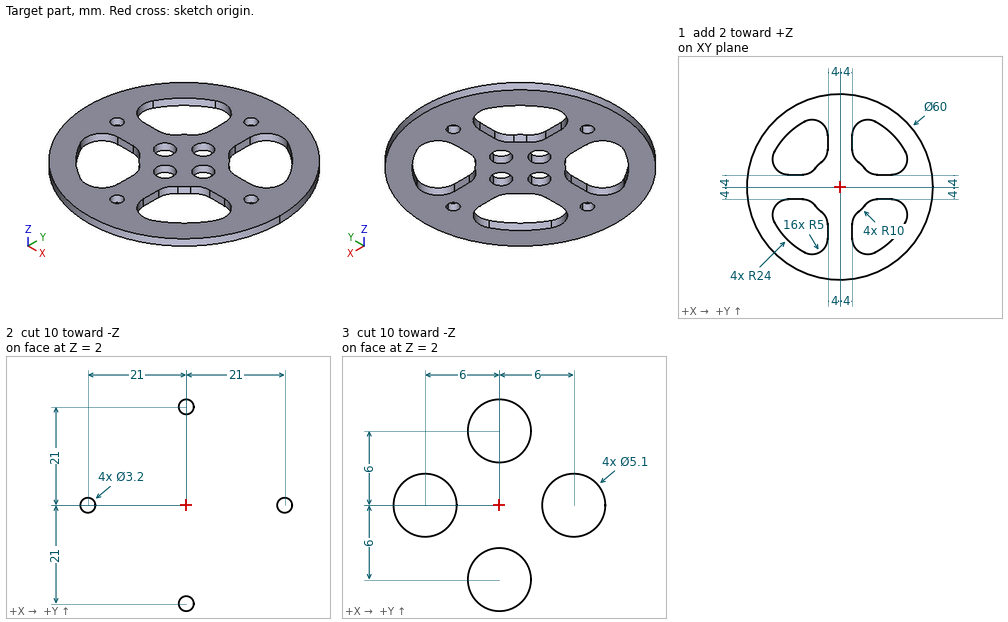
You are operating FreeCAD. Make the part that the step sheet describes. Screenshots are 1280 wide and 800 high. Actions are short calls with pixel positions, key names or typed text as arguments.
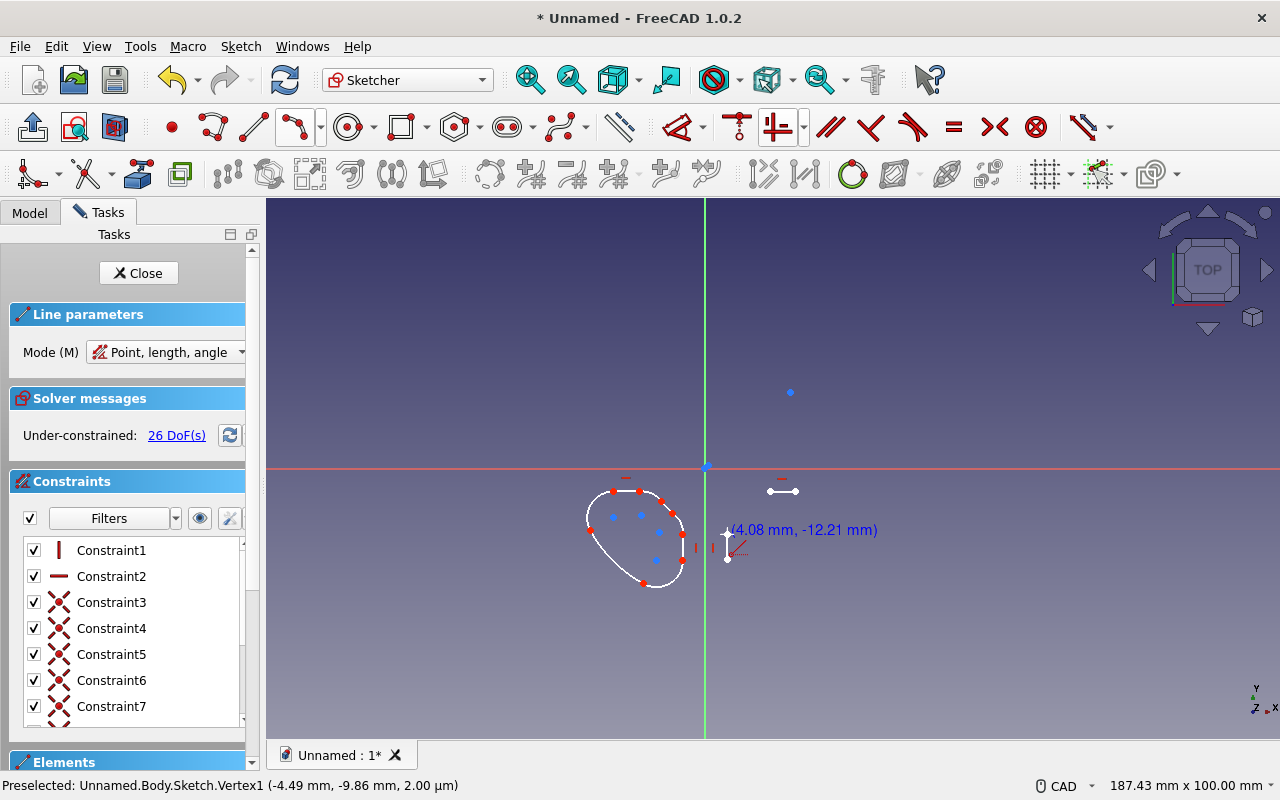
click(294, 128)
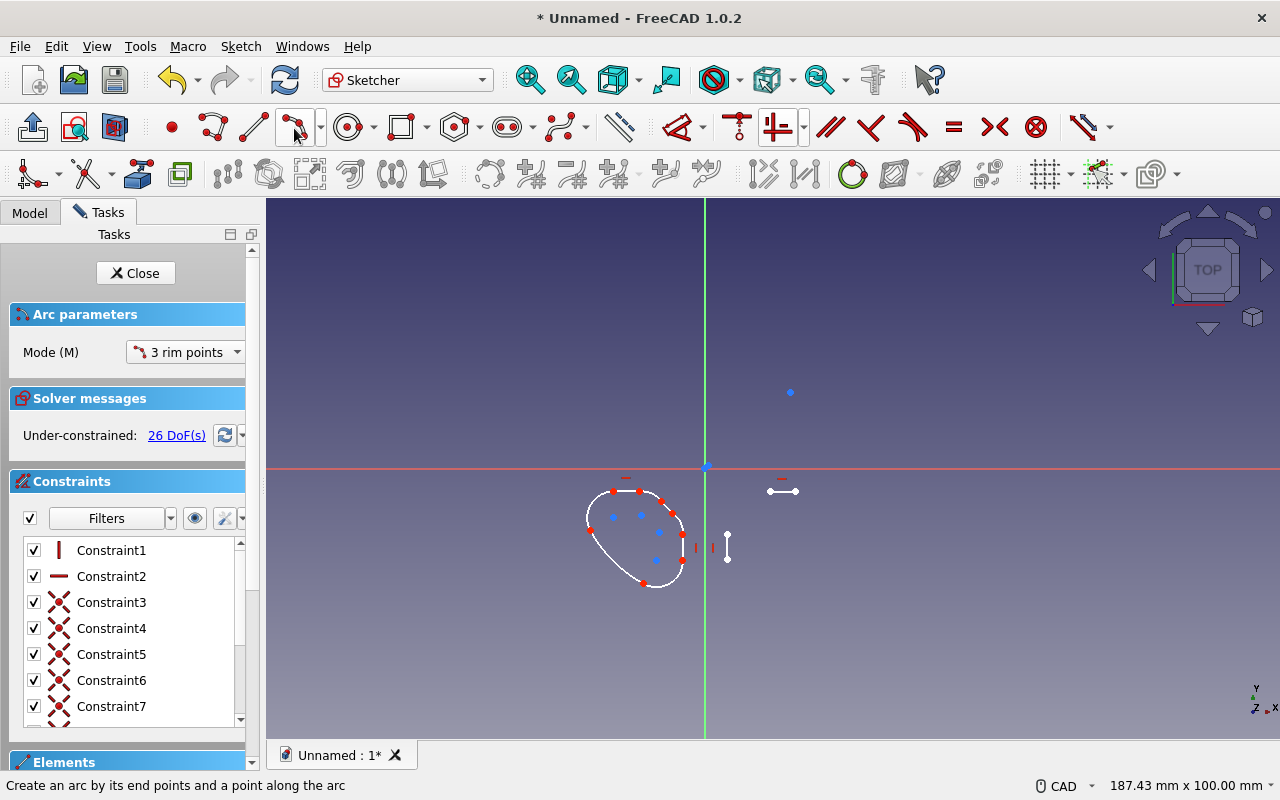
scroll(795, 491, up, 2)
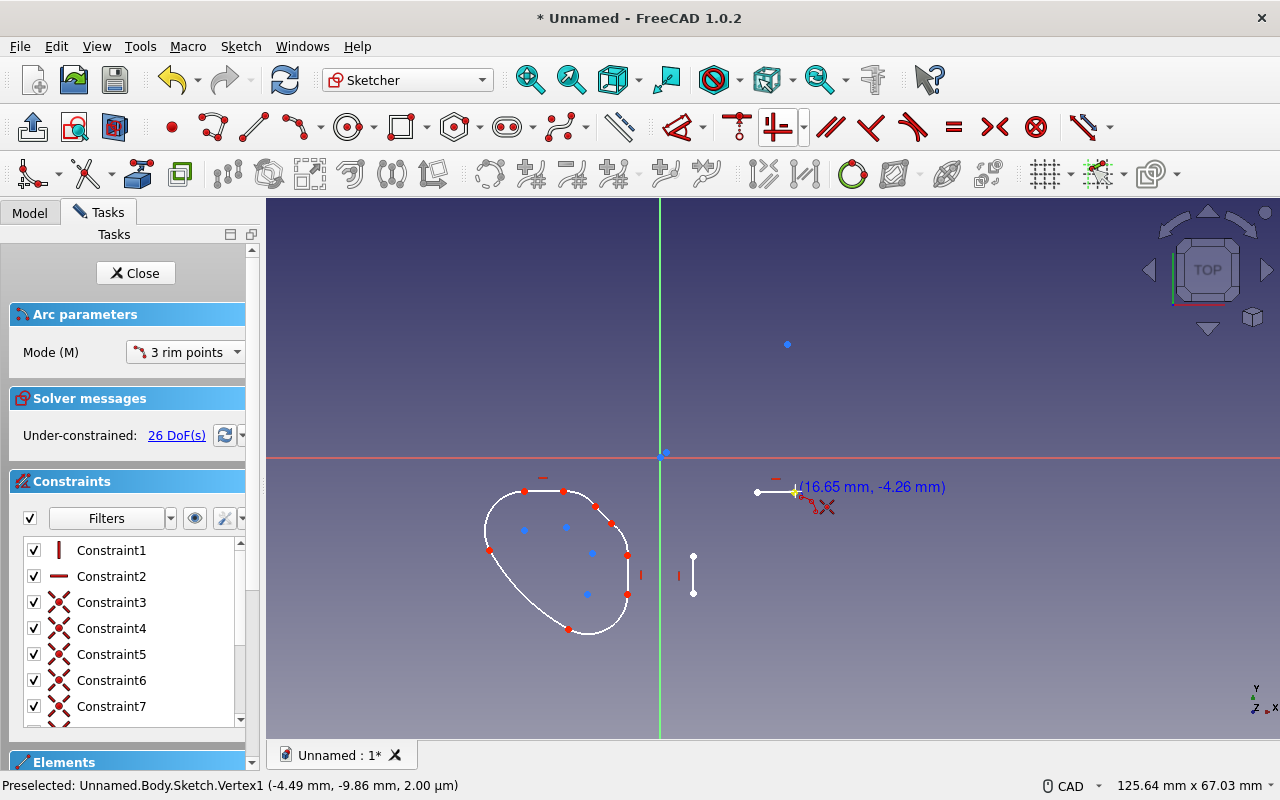
click(795, 492)
click(831, 550)
click(830, 510)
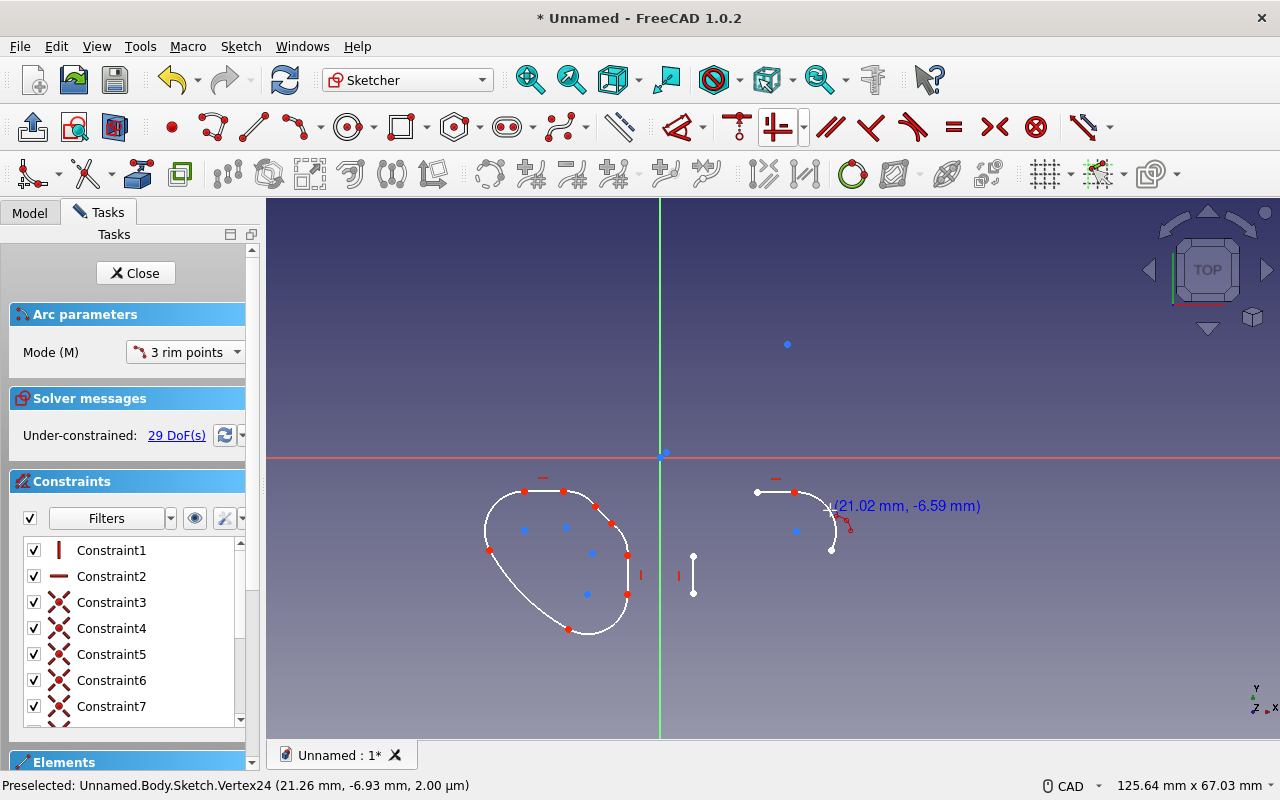
click(831, 551)
click(752, 628)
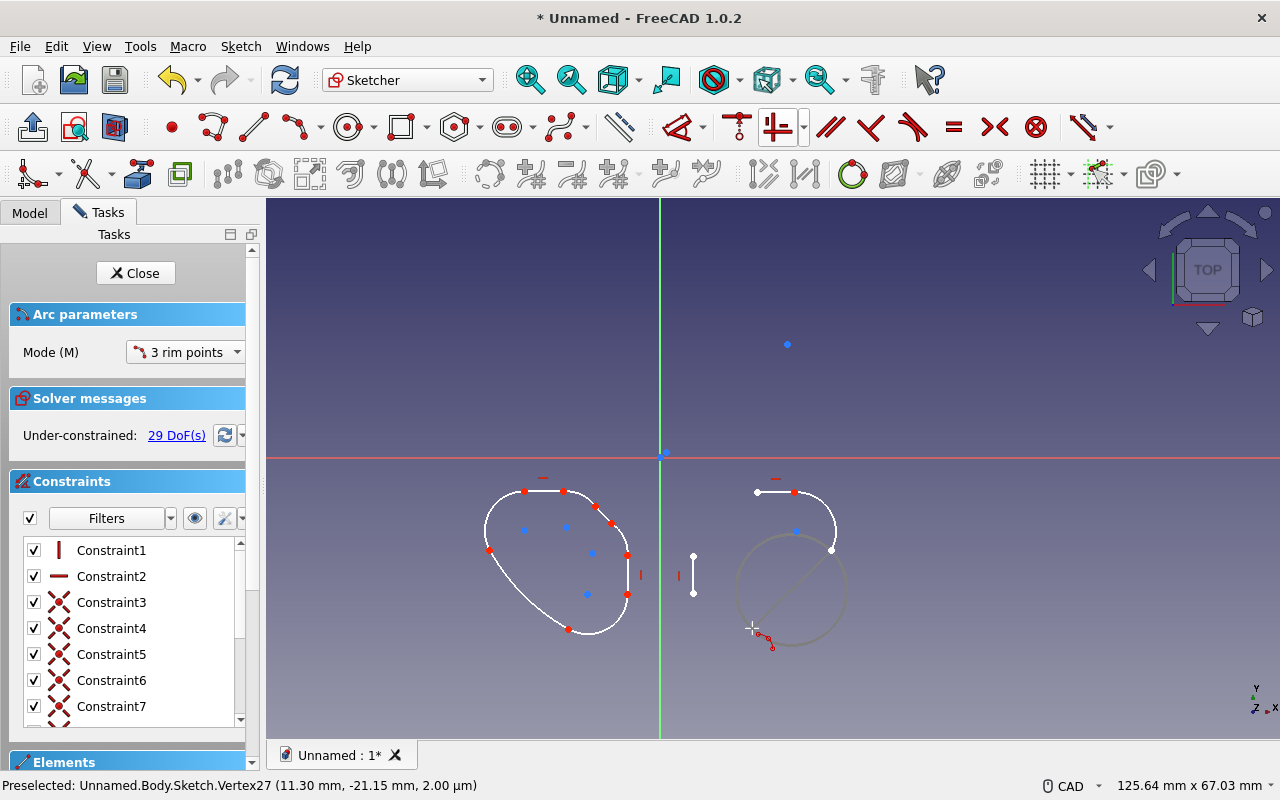
scroll(797, 595, up, 4)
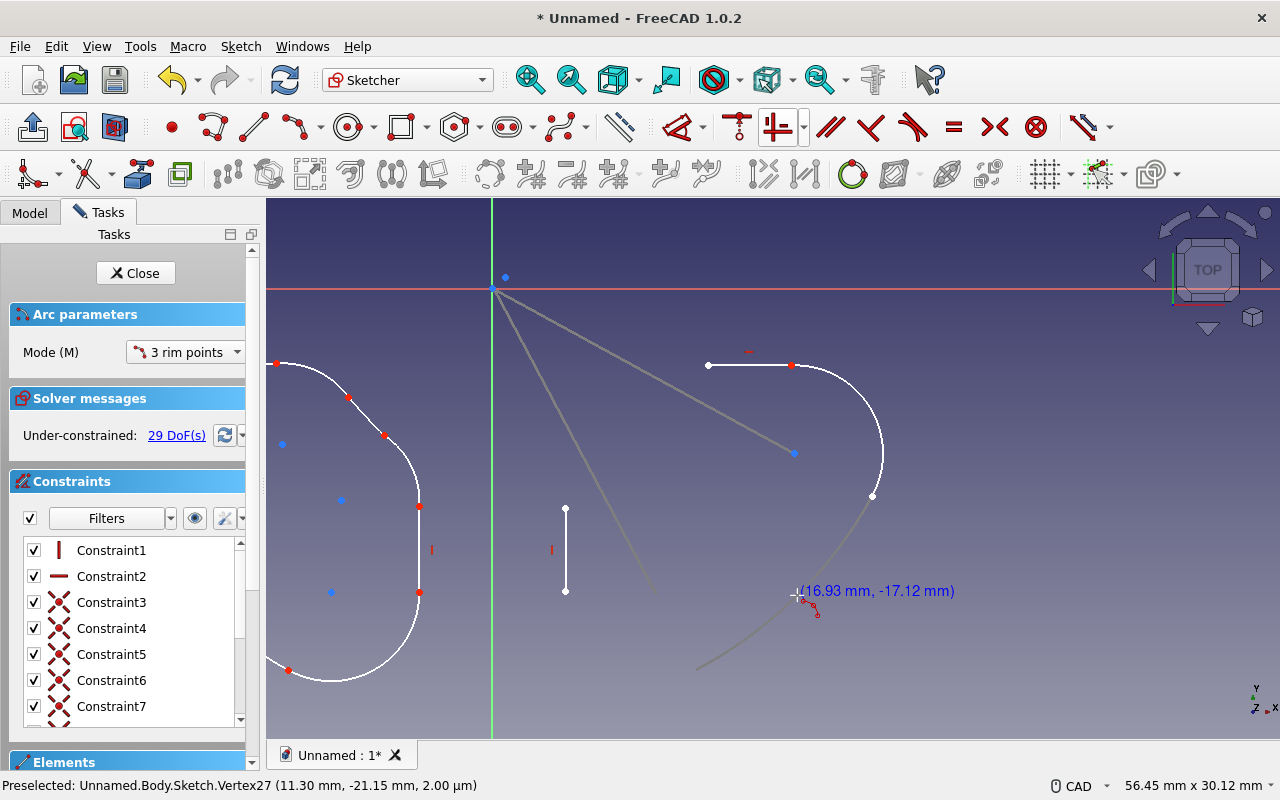
click(797, 594)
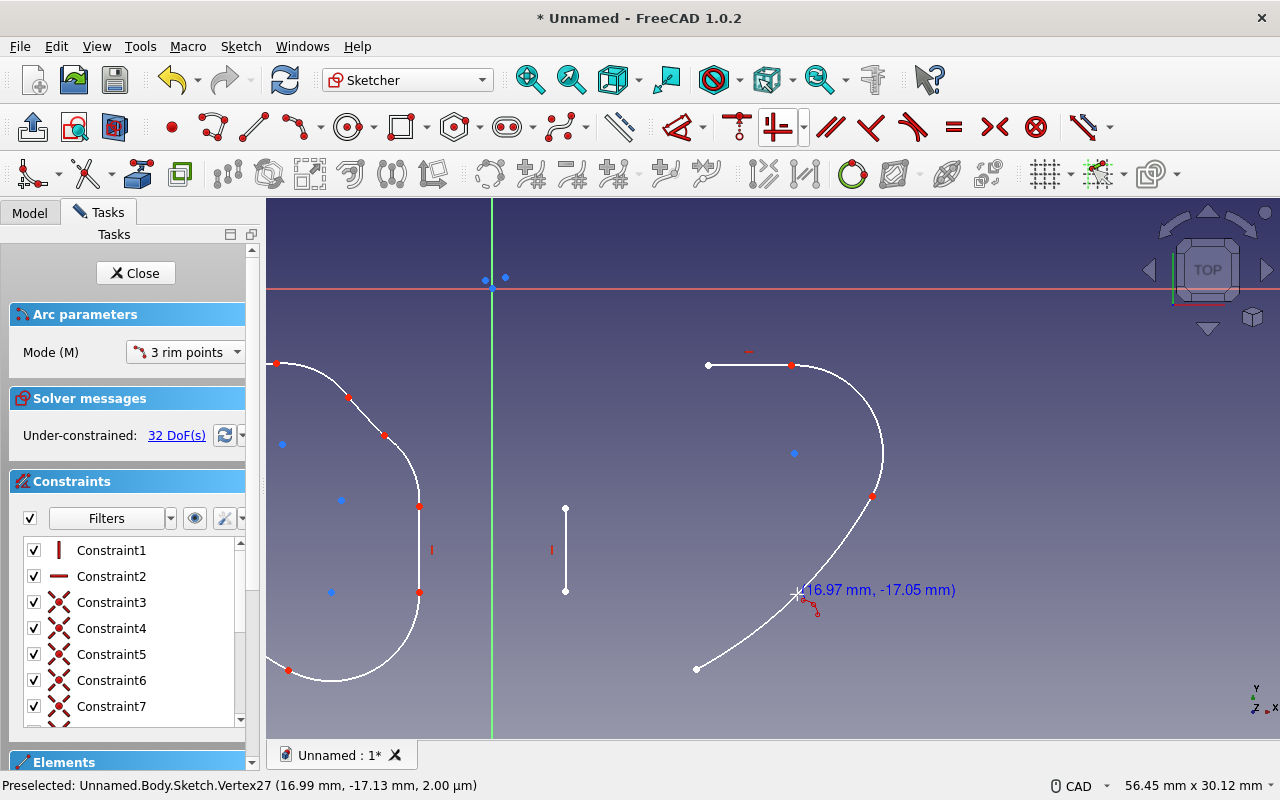
click(696, 670)
click(566, 591)
click(608, 666)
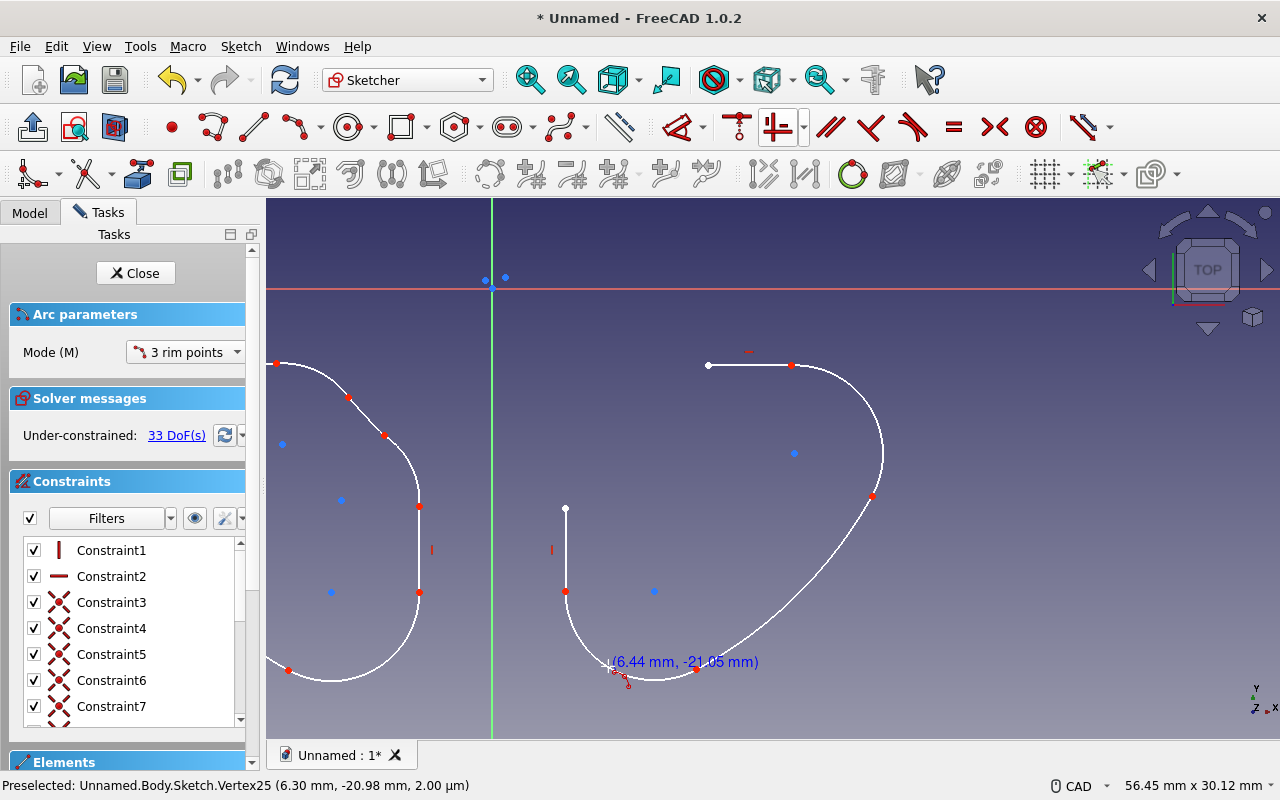
click(566, 508)
click(600, 433)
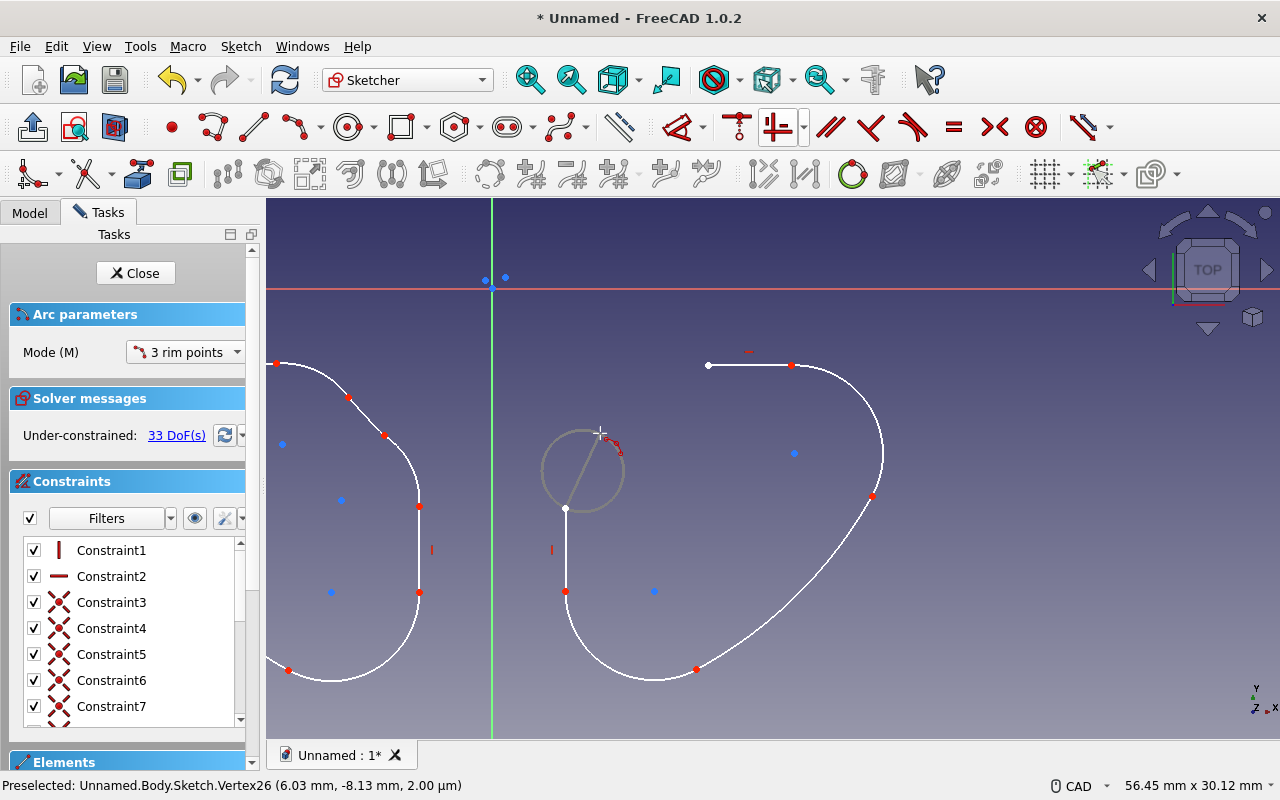
scroll(574, 464, up, 3)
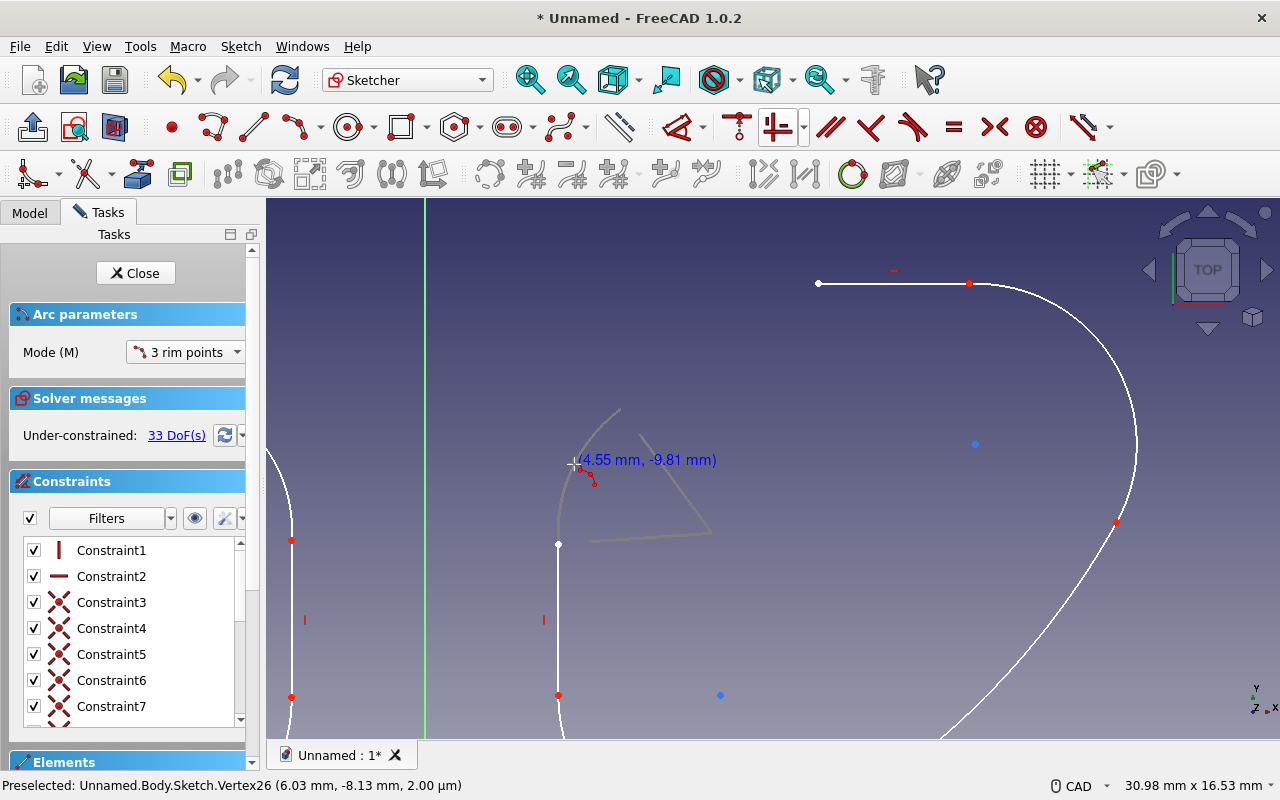
click(573, 464)